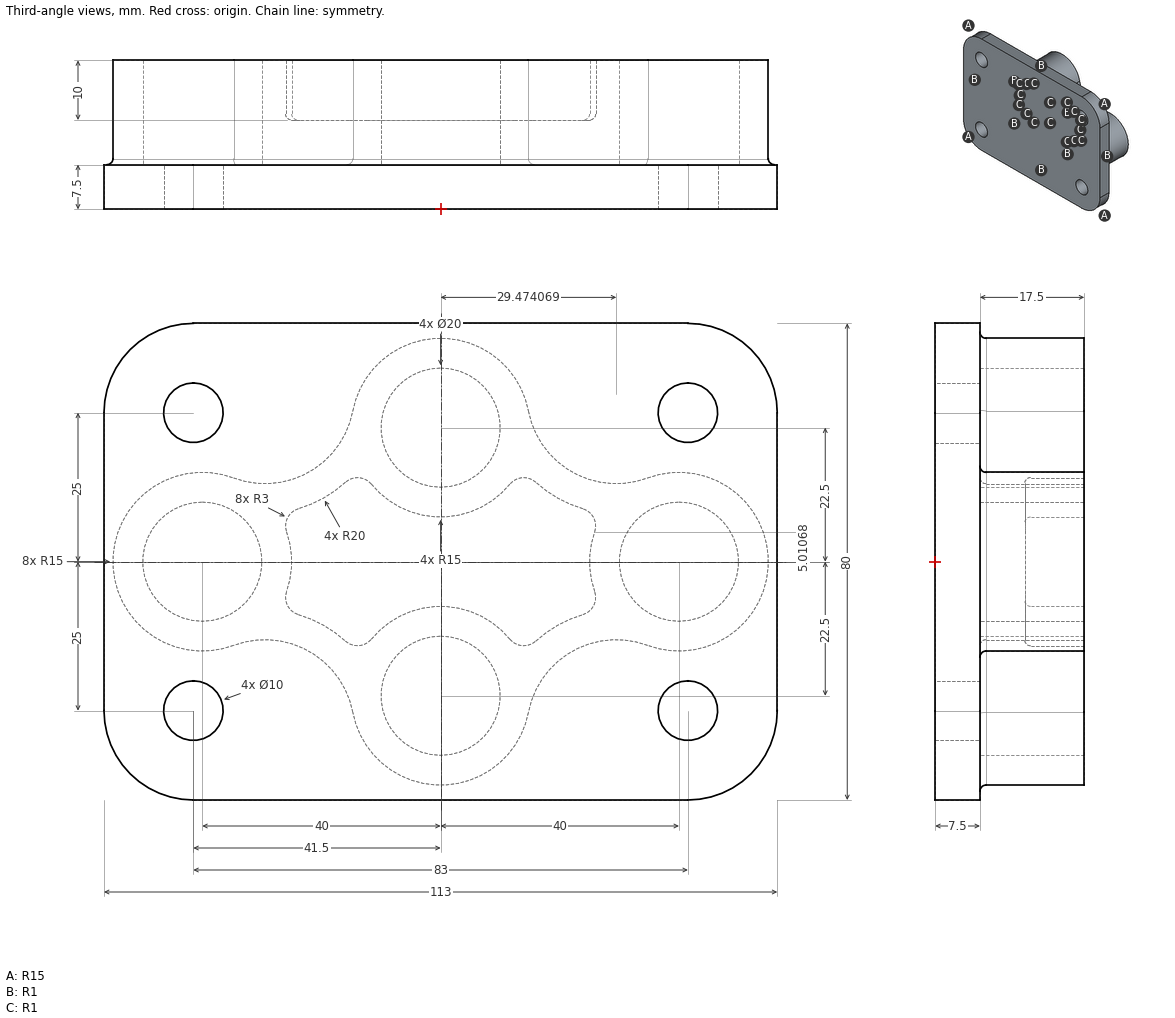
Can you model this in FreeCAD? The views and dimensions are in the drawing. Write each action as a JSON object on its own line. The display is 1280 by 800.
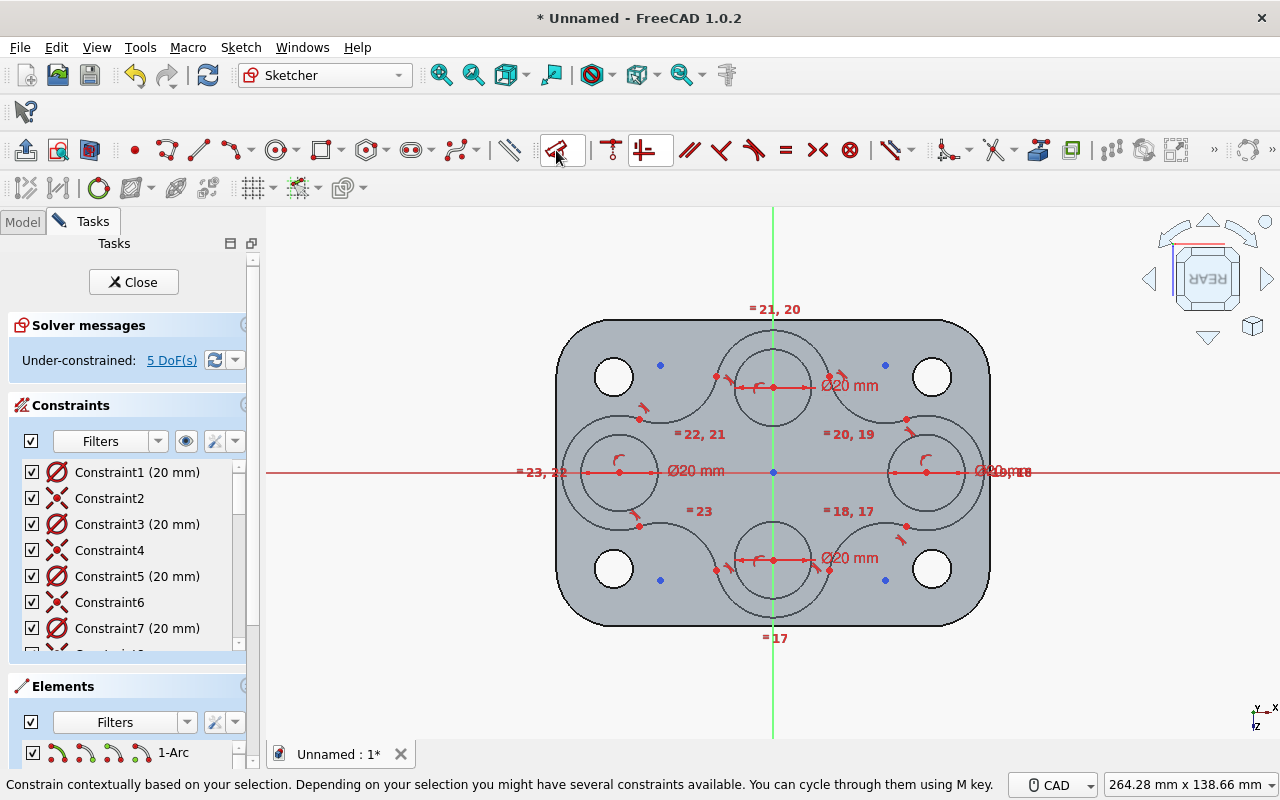
{"action": "left_click", "coordinate": [743, 609]}
{"action": "left_click", "coordinate": [726, 636]}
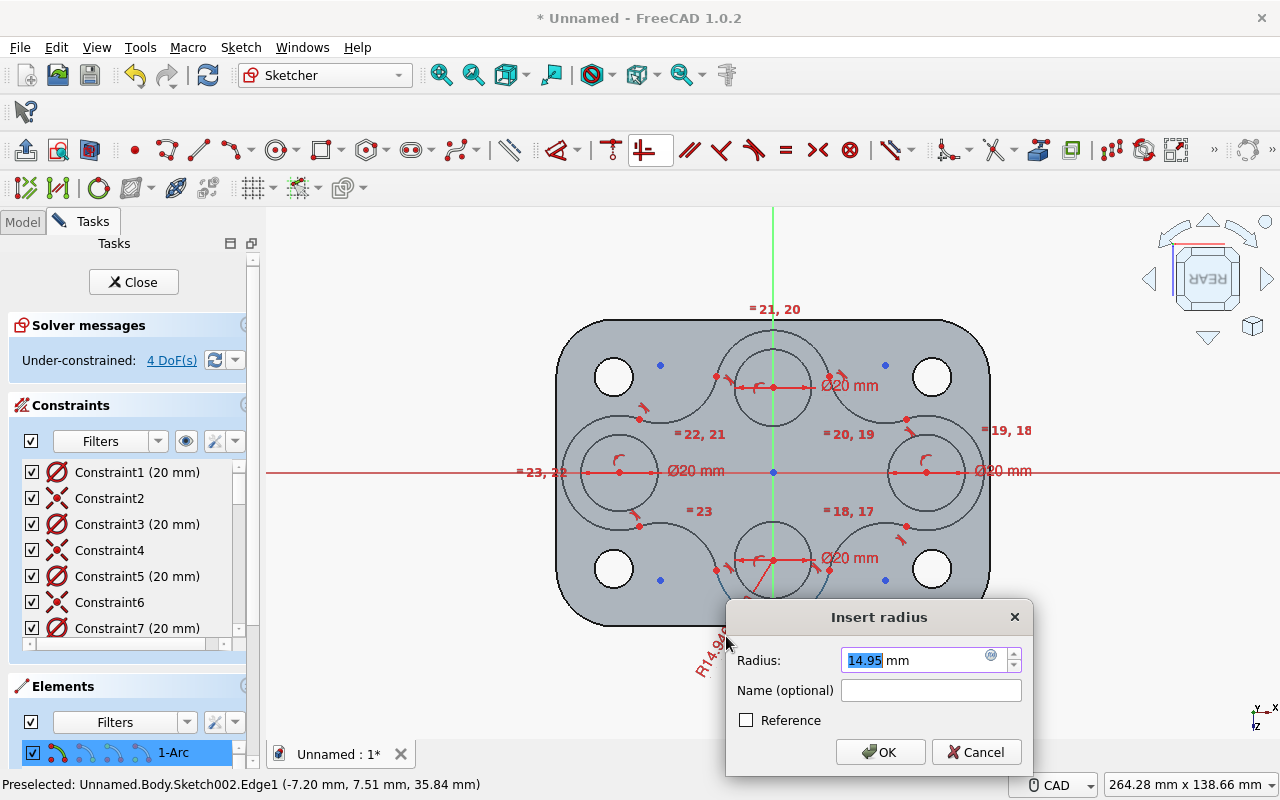
{"action": "type", "text": "15"}
{"action": "key", "text": "Return"}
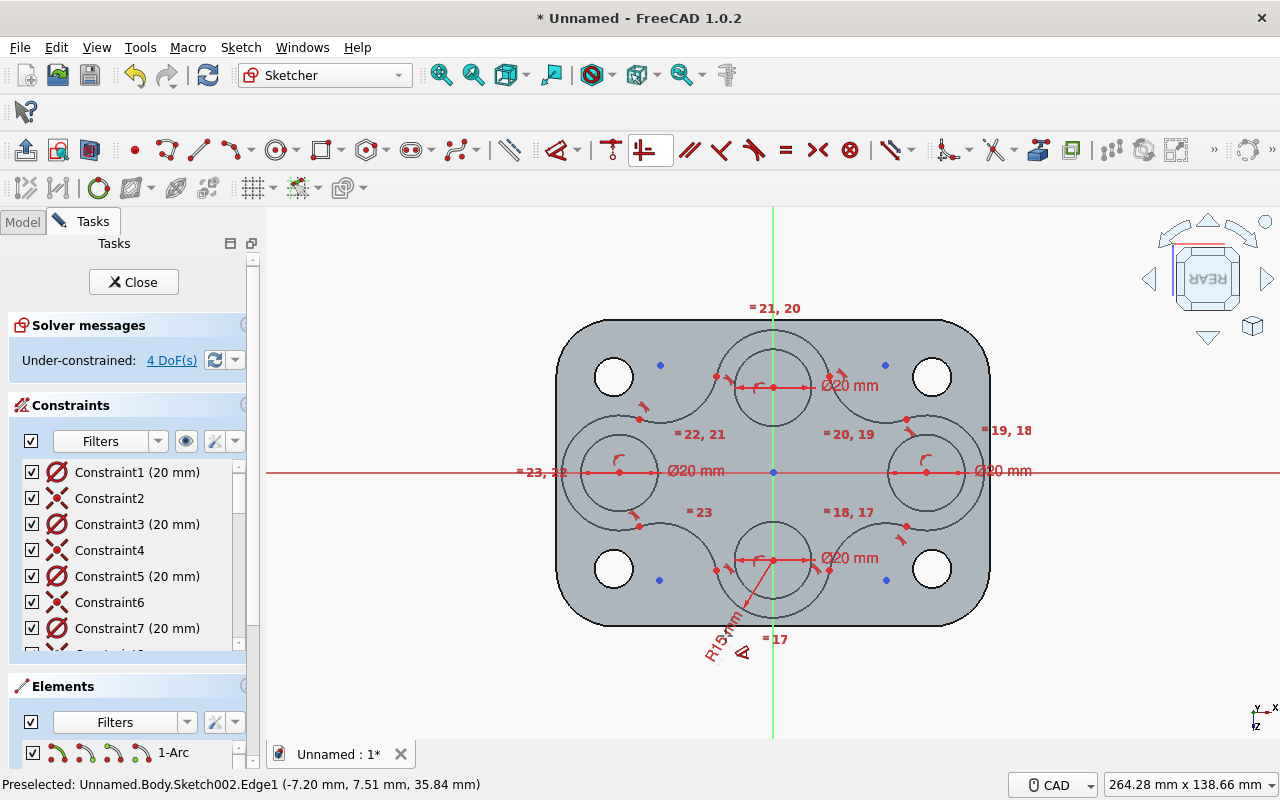
{"action": "left_click", "coordinate": [619, 473]}
{"action": "left_click", "coordinate": [696, 507]}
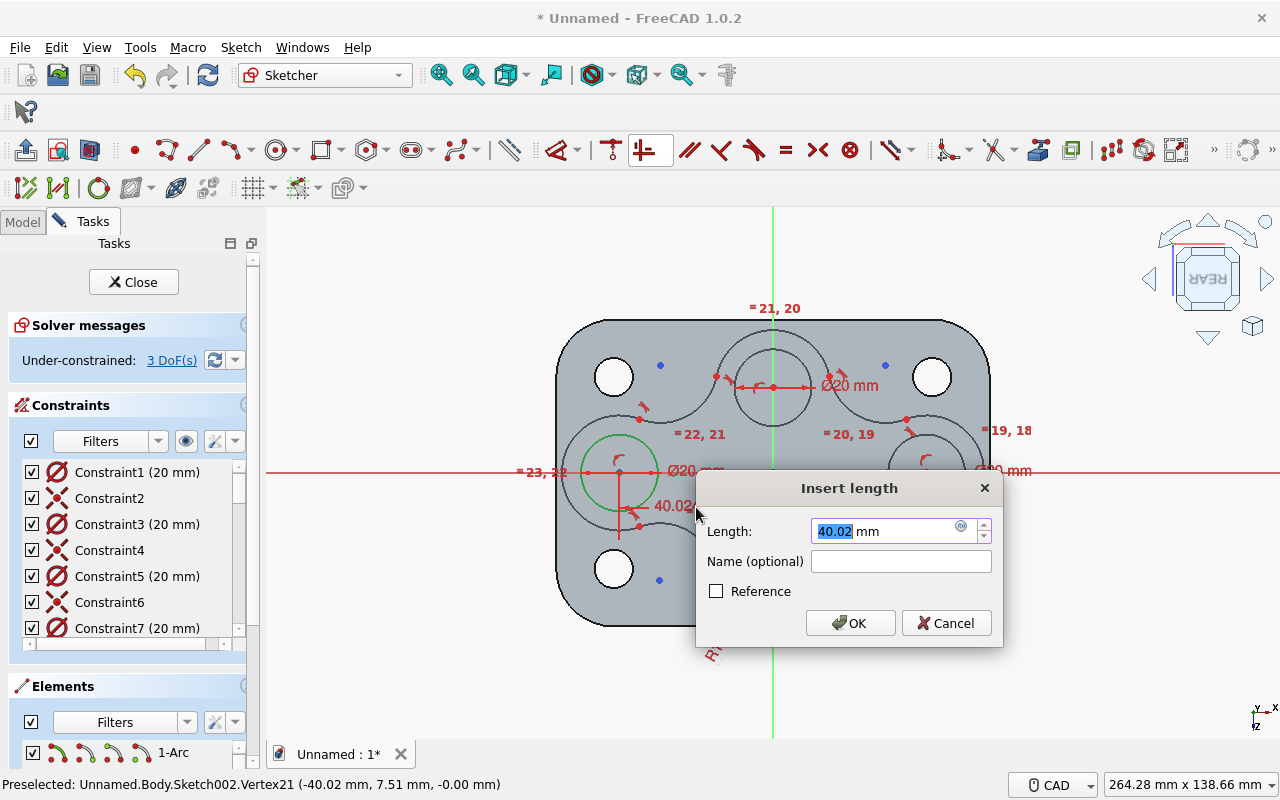
{"action": "type", "text": "40"}
{"action": "key", "text": "Return"}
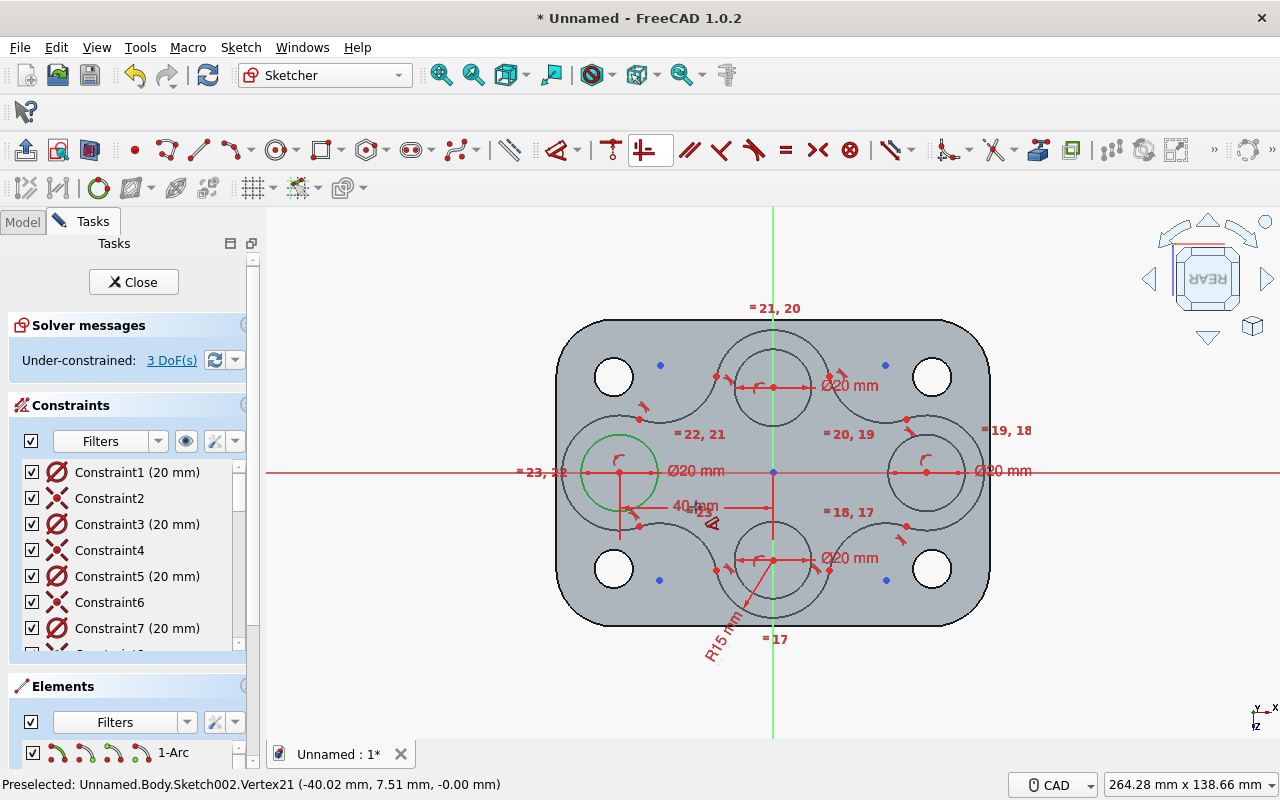
{"action": "left_click", "coordinate": [927, 473]}
{"action": "left_click", "coordinate": [850, 507]}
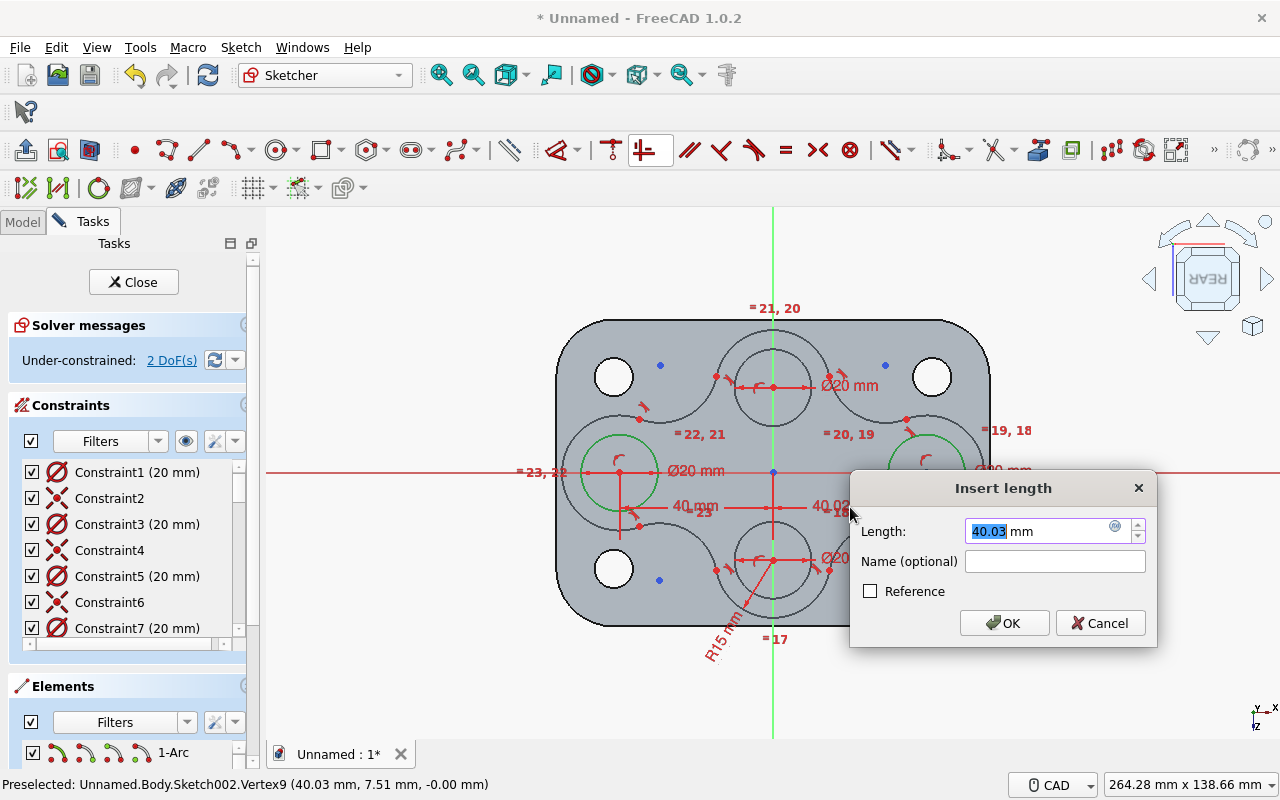
{"action": "type", "text": "40"}
{"action": "key", "text": "Return"}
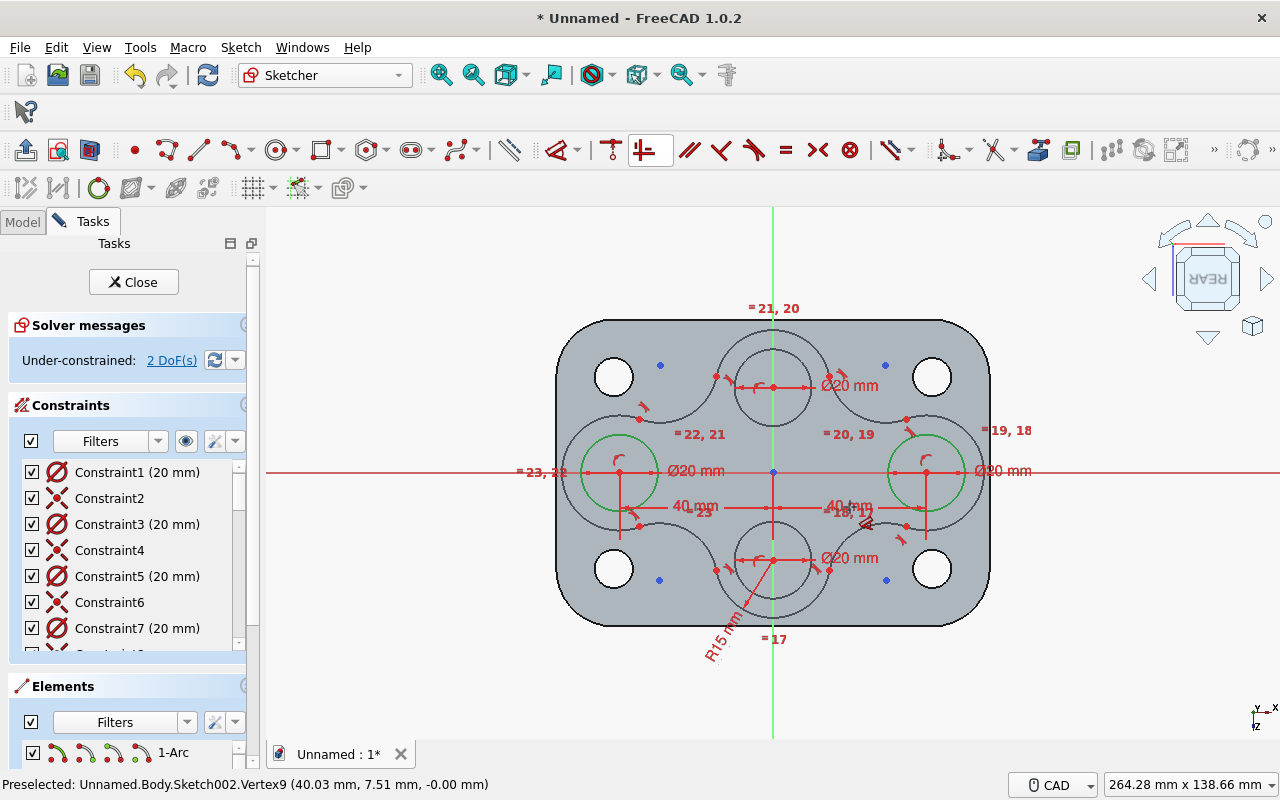
{"action": "left_click", "coordinate": [773, 560]}
{"action": "left_click", "coordinate": [807, 486]}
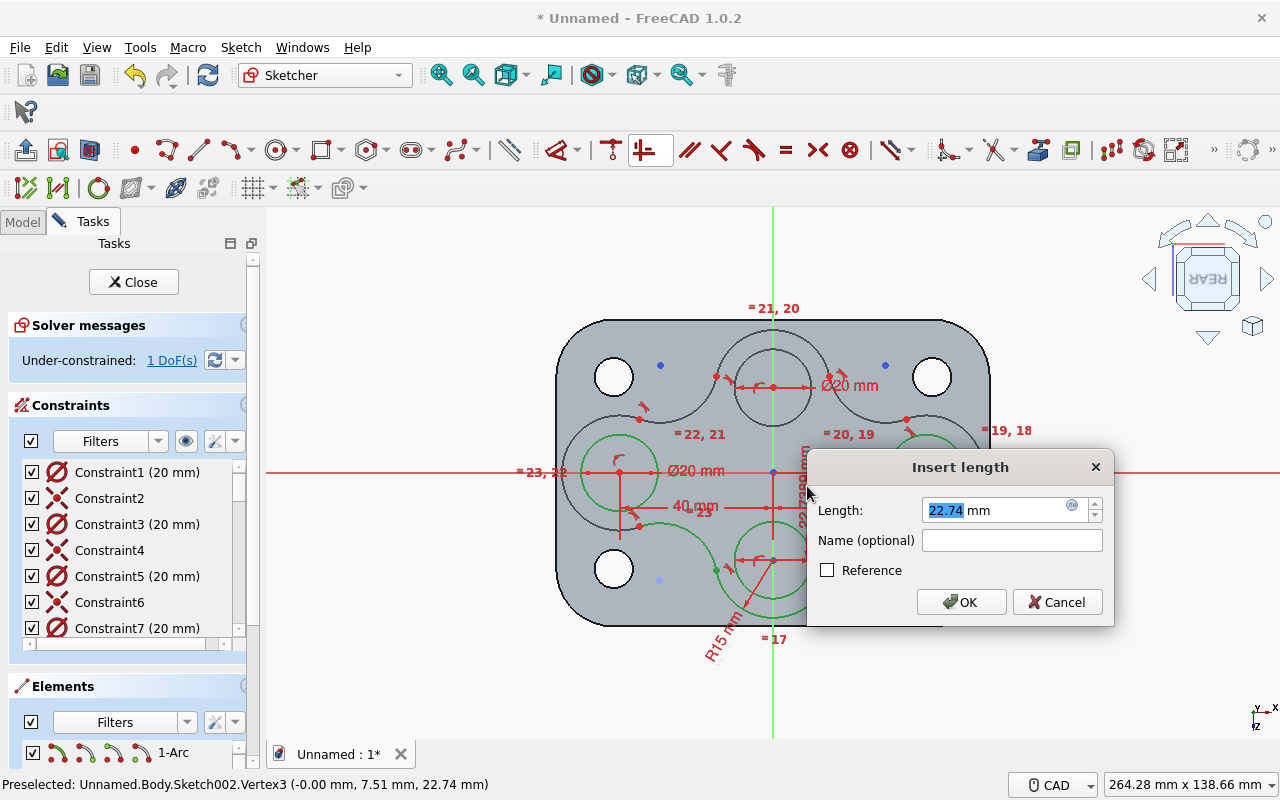
{"action": "type", "text": "22.5"}
{"action": "key", "text": "Return"}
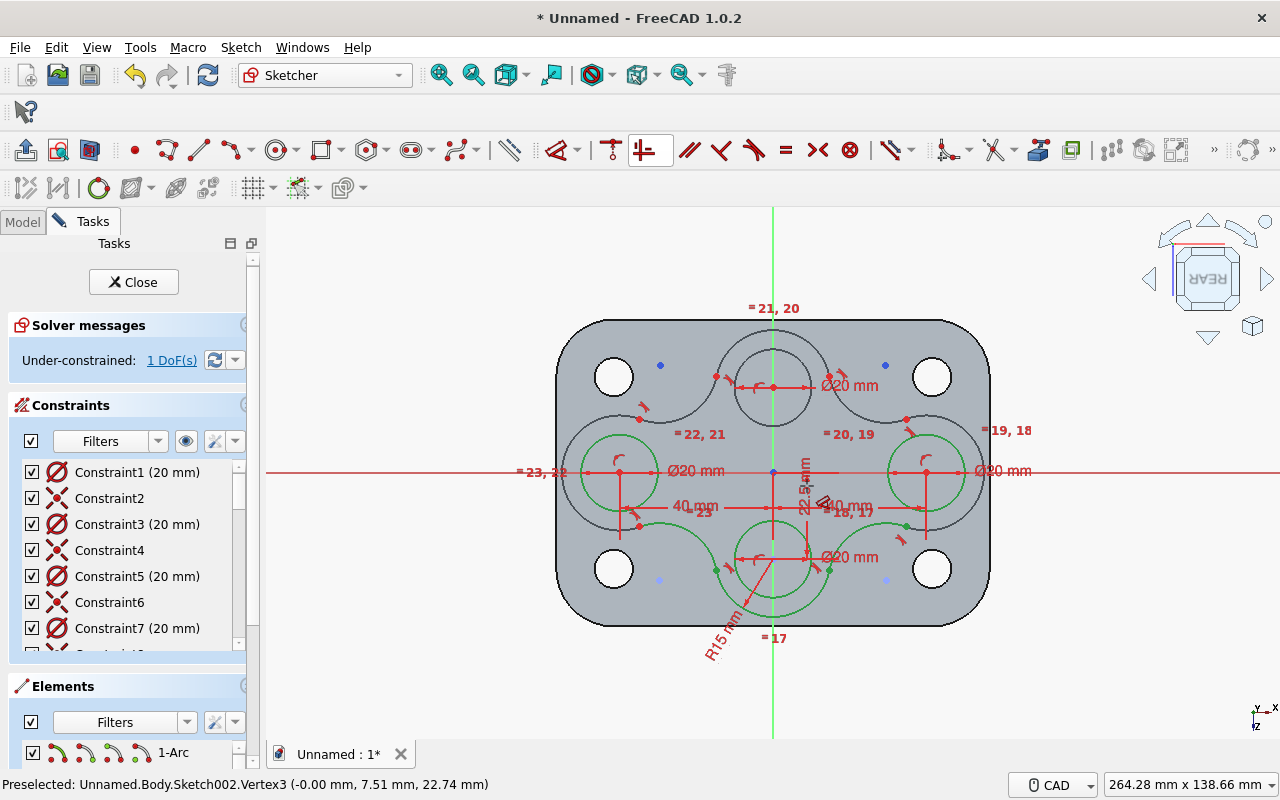
{"action": "left_click", "coordinate": [773, 388]}
{"action": "left_click", "coordinate": [807, 430]}